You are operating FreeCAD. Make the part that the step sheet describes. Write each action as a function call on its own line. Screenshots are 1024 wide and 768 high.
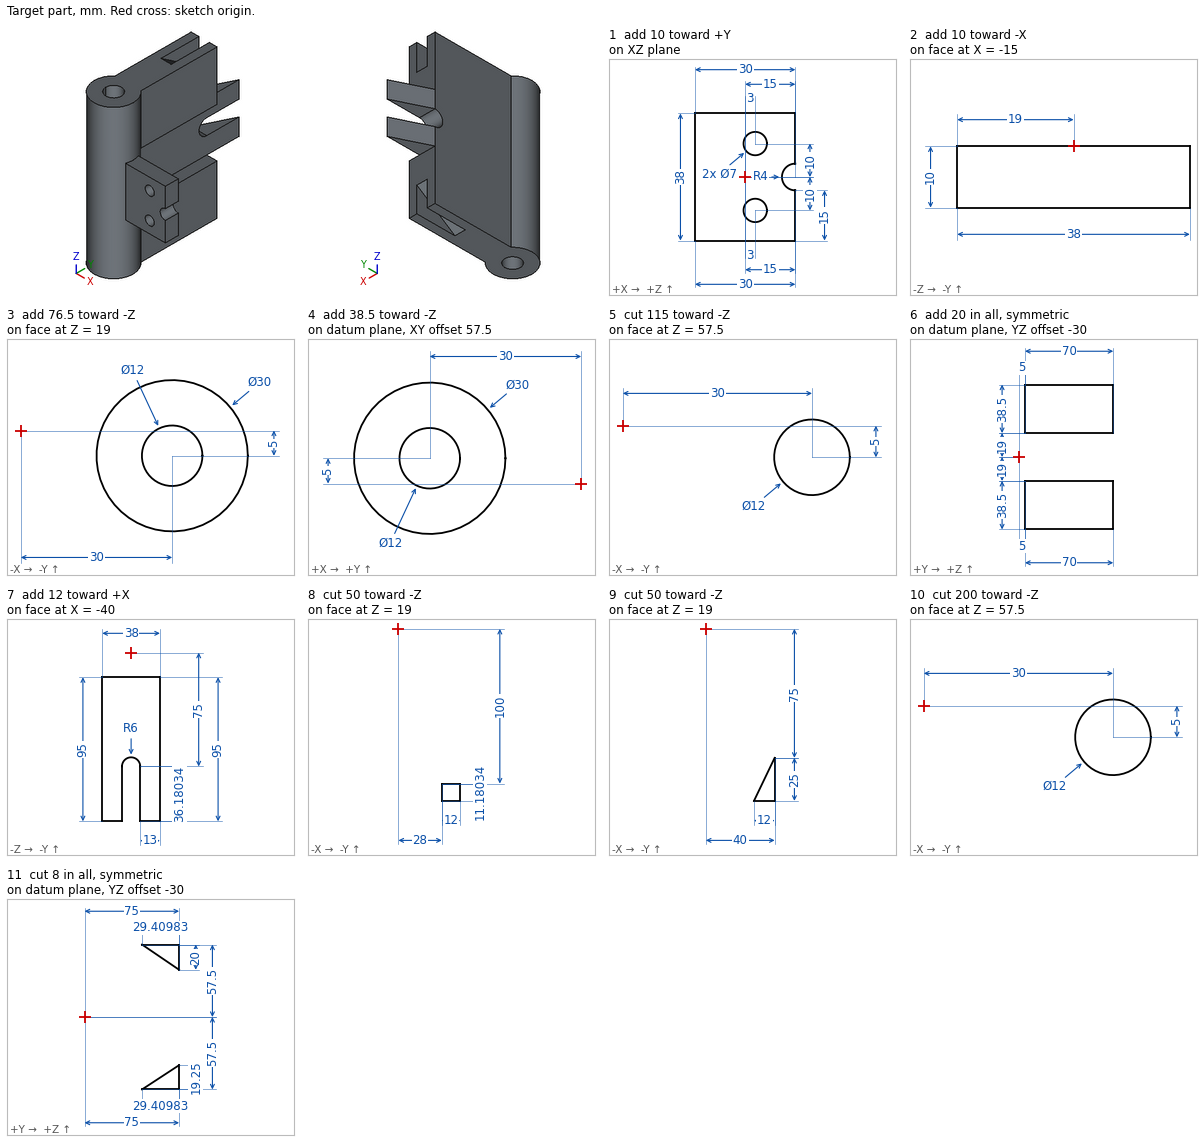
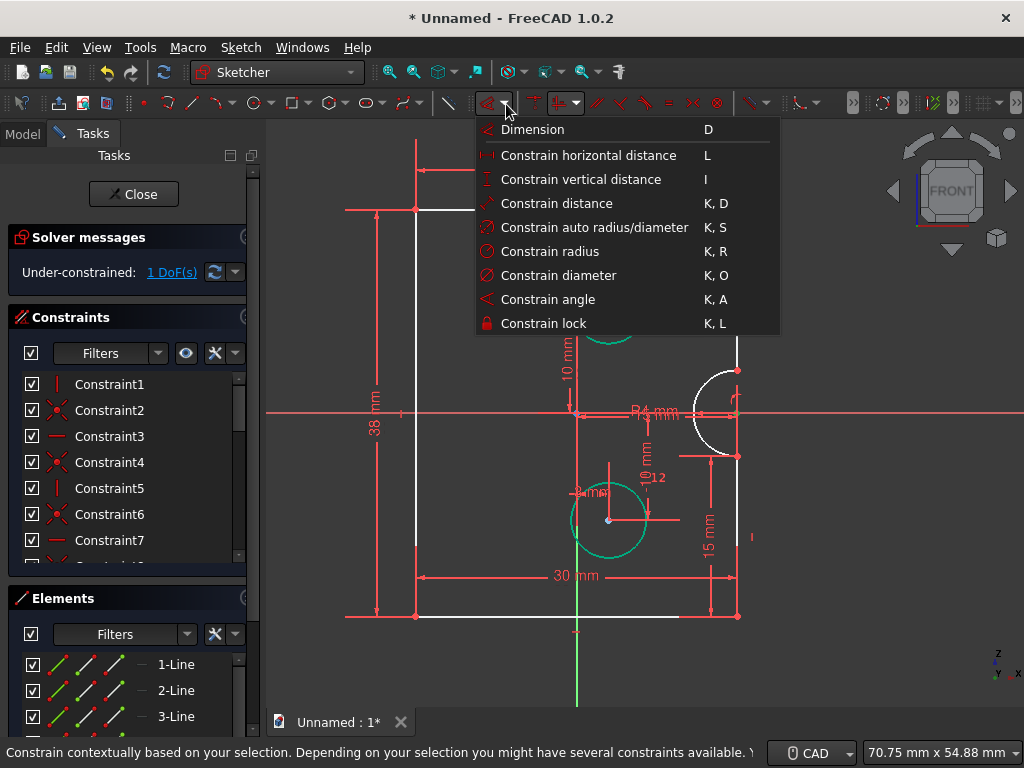
click(628, 155)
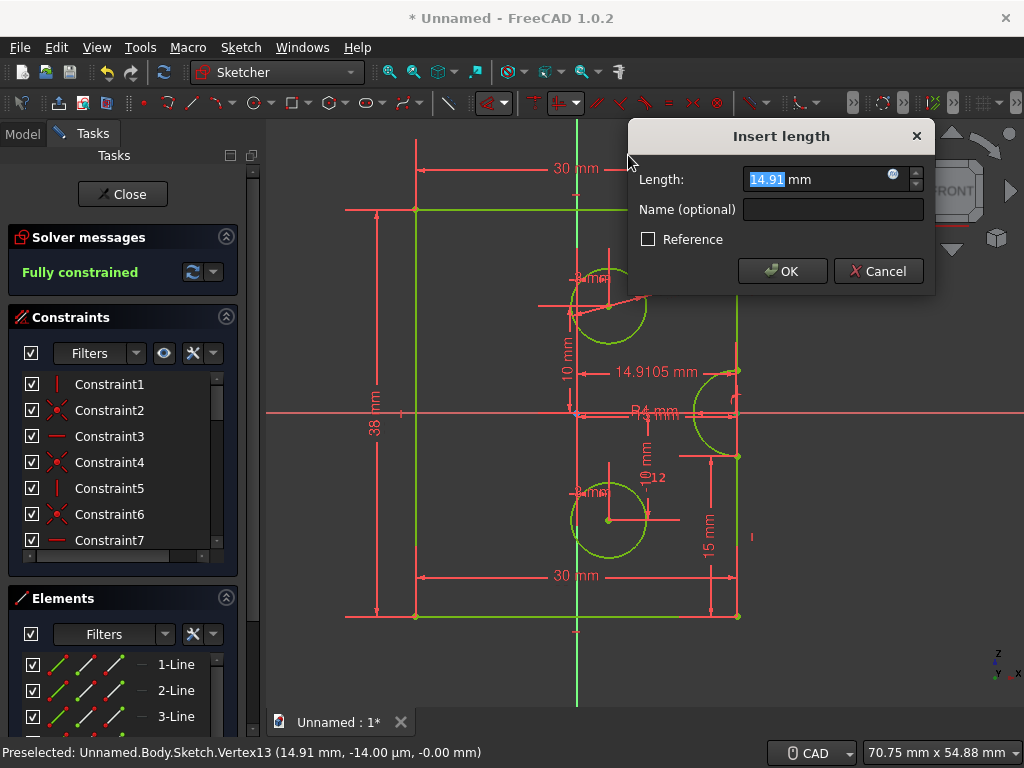
text(15)
key(Return)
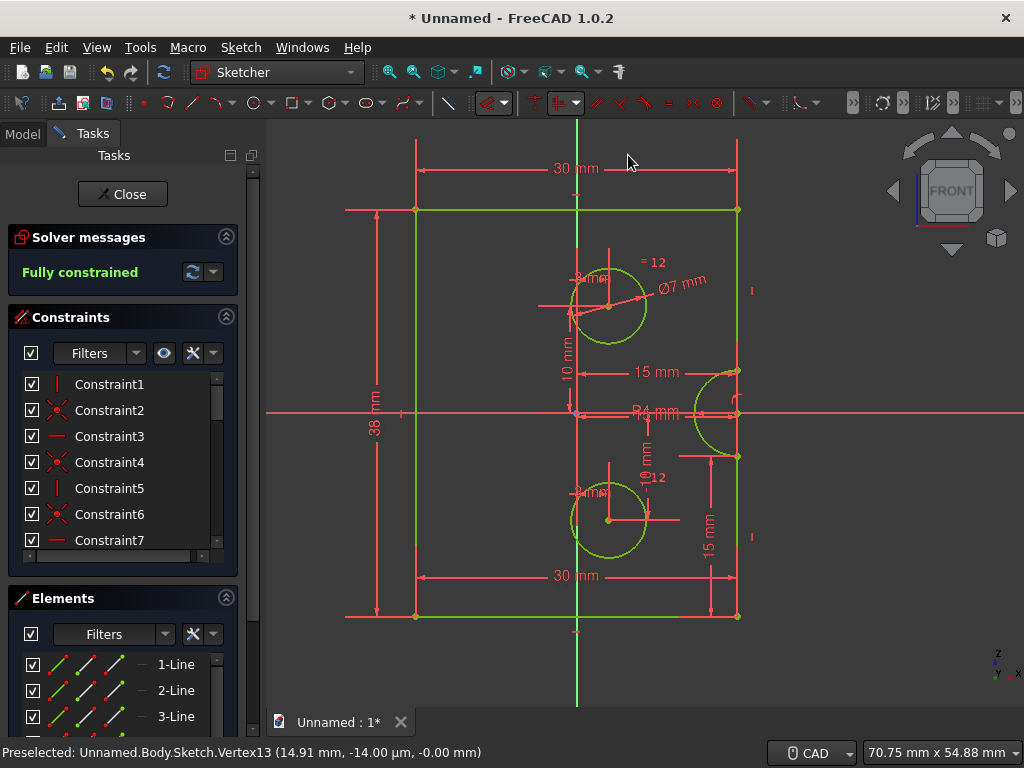
click(123, 194)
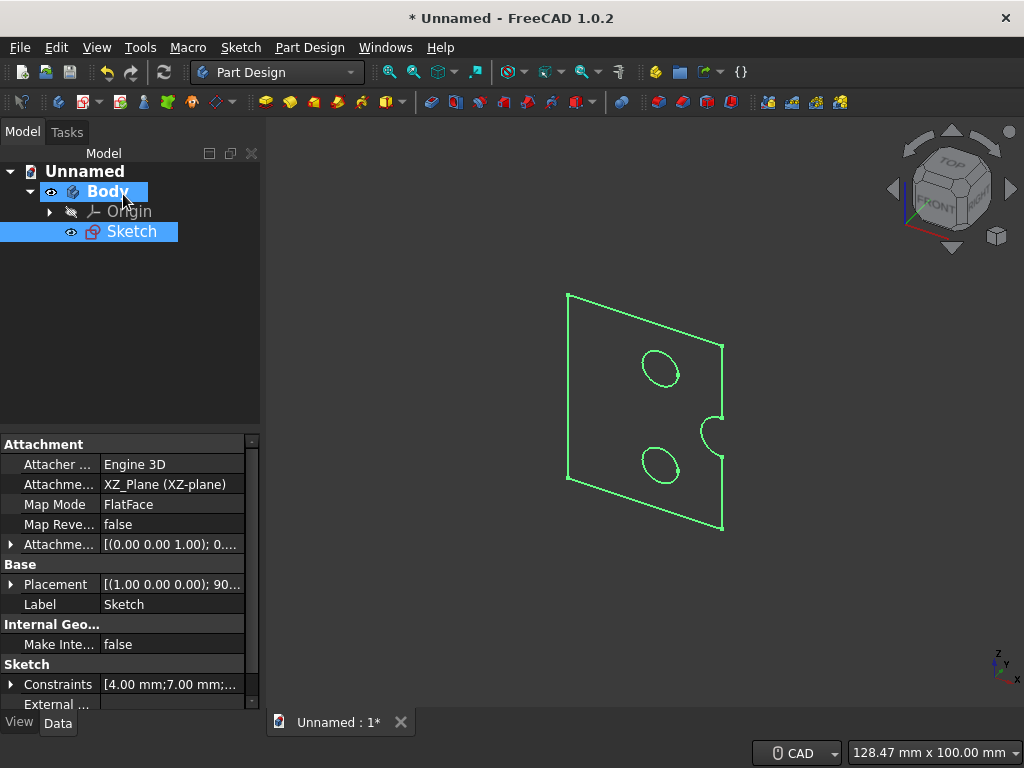
click(266, 102)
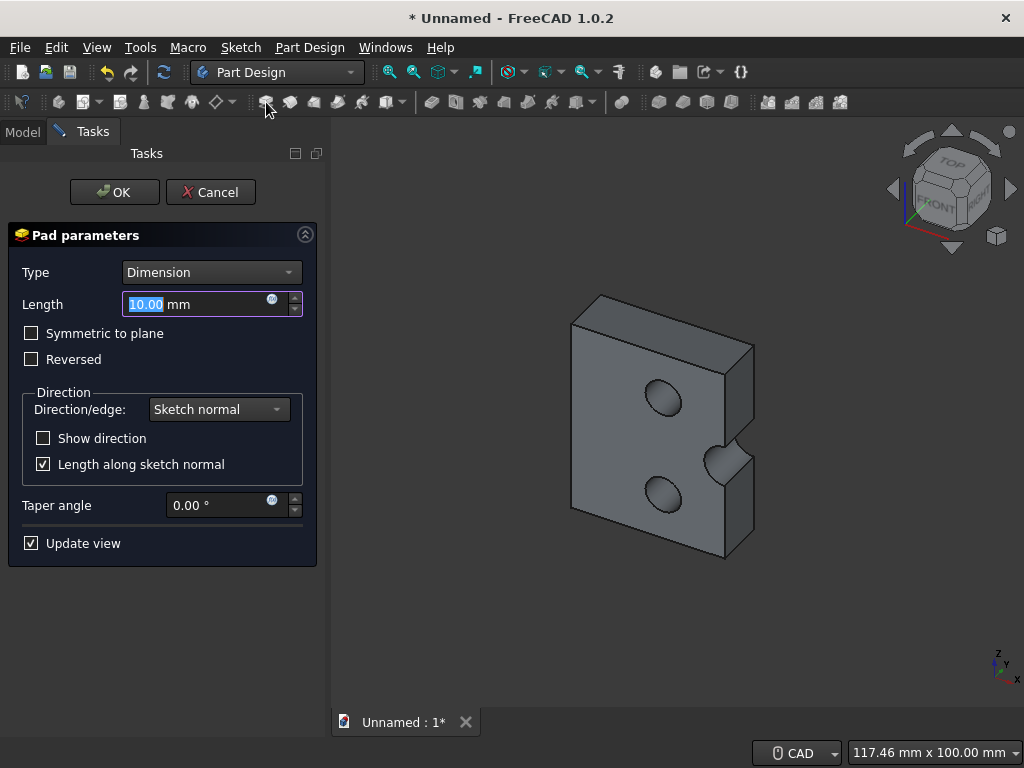
text(10)
key(Tab)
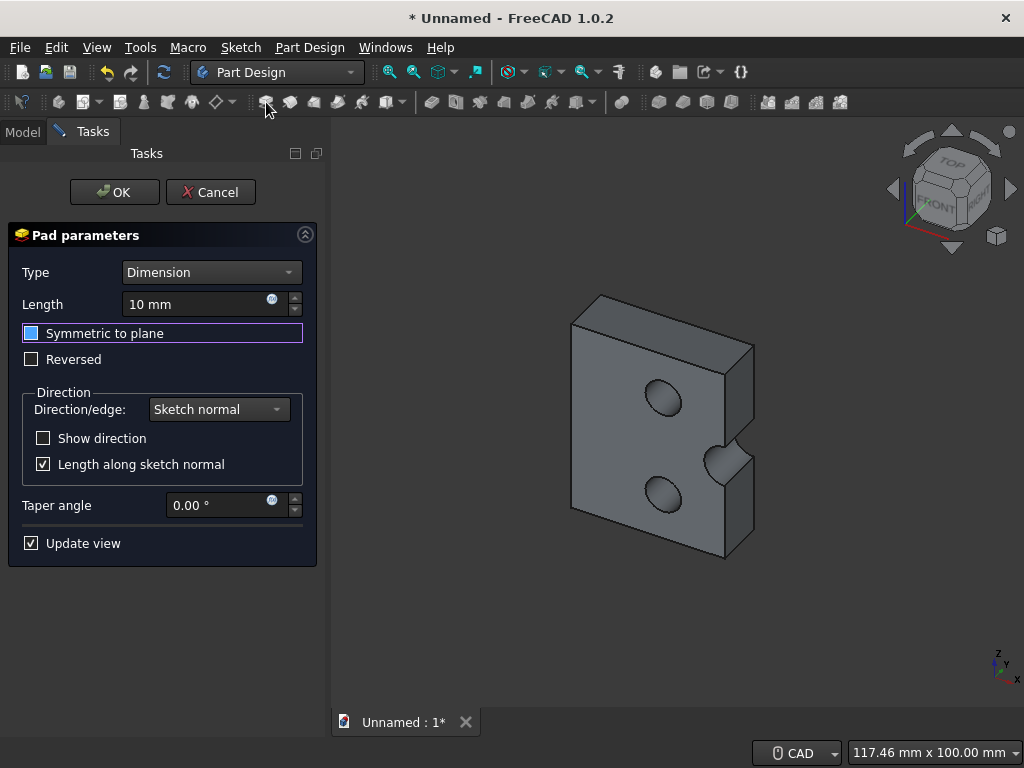
click(30, 359)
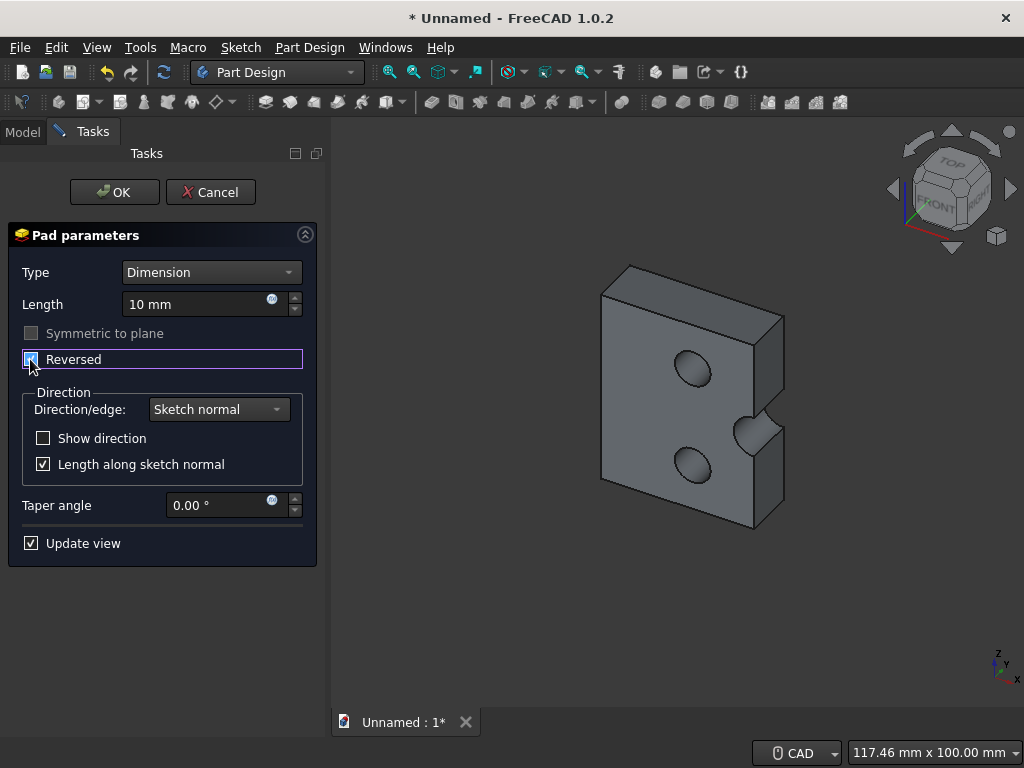
click(115, 192)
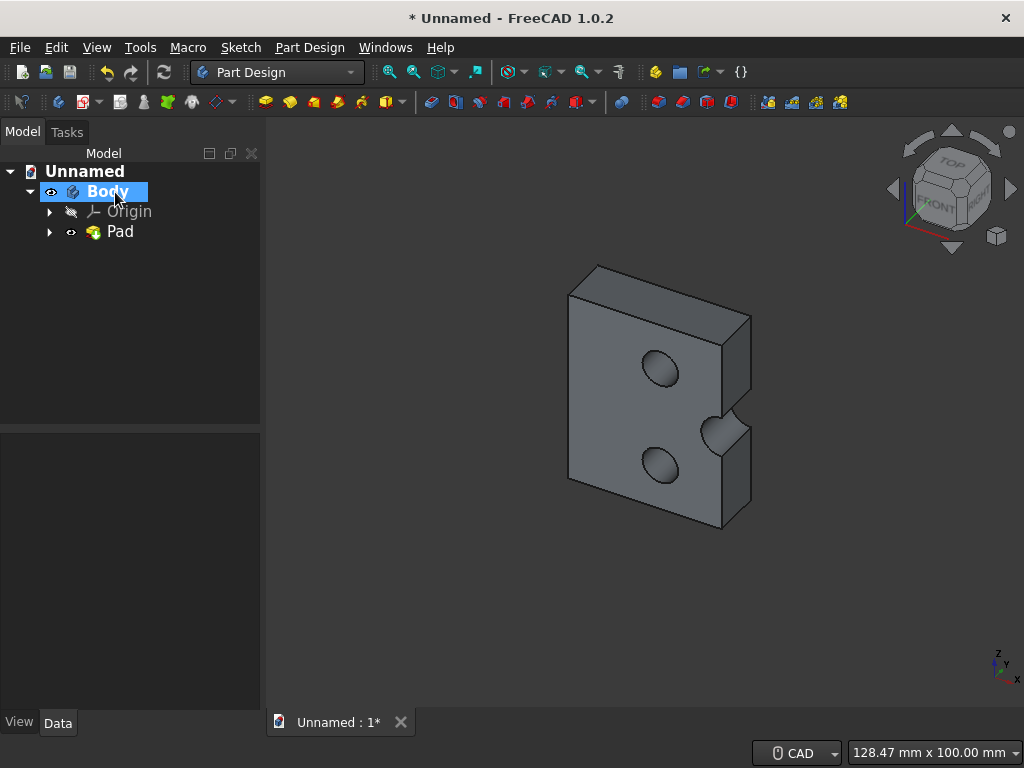
key(v)
key(f)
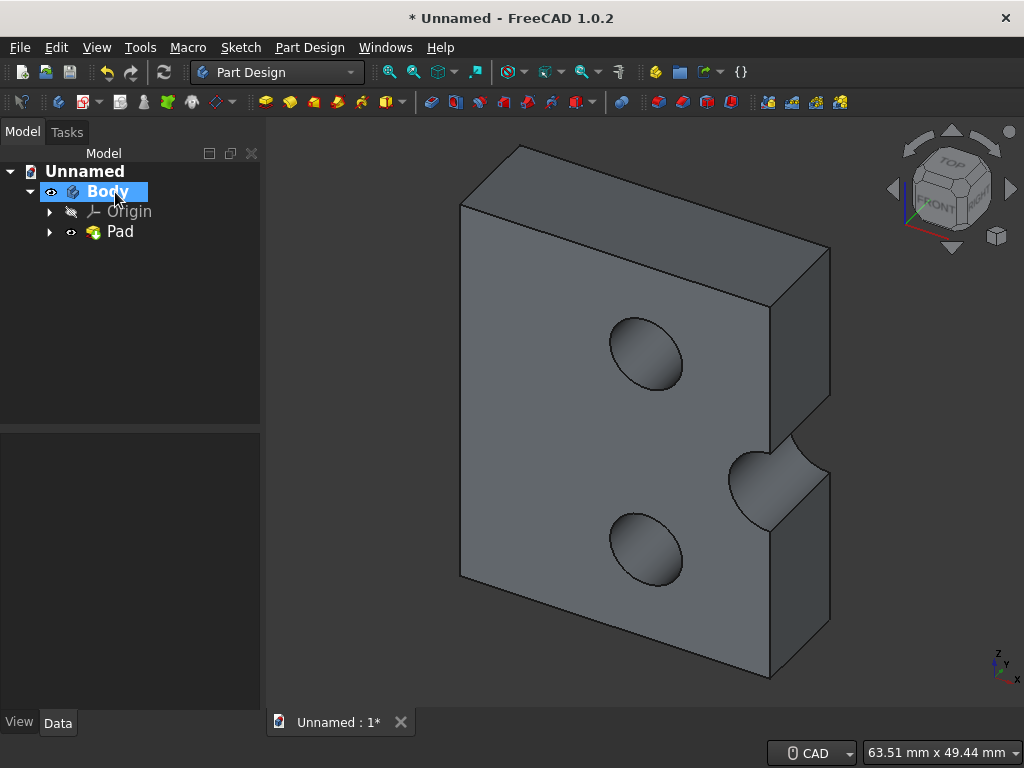
key(6)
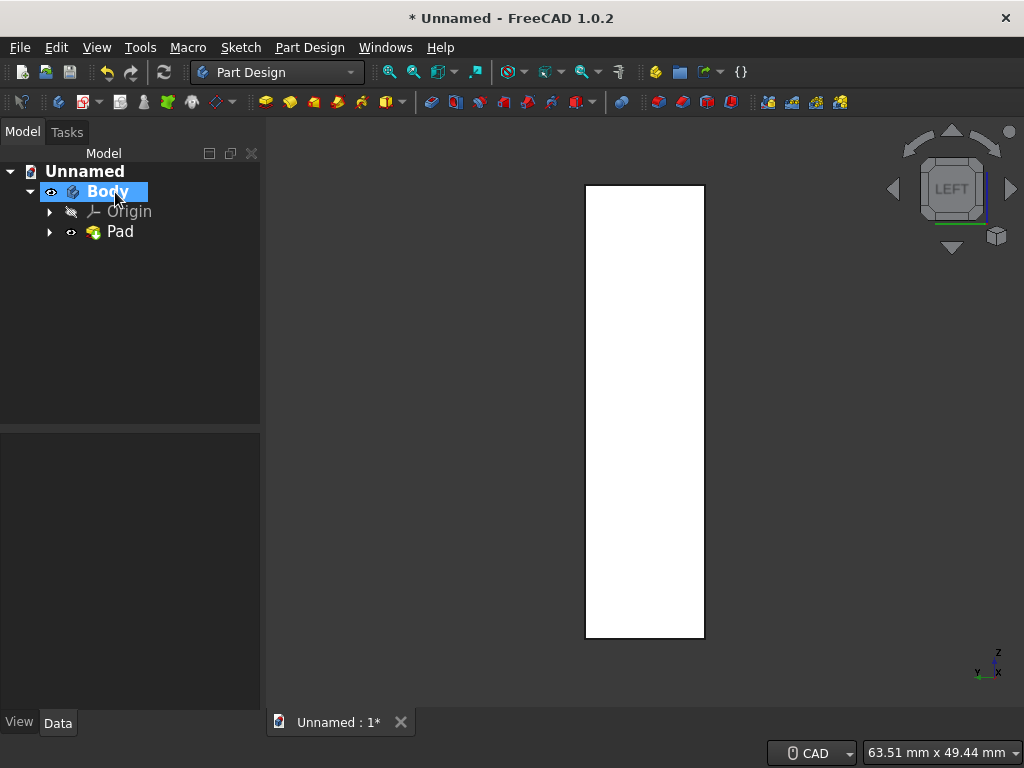
click(645, 346)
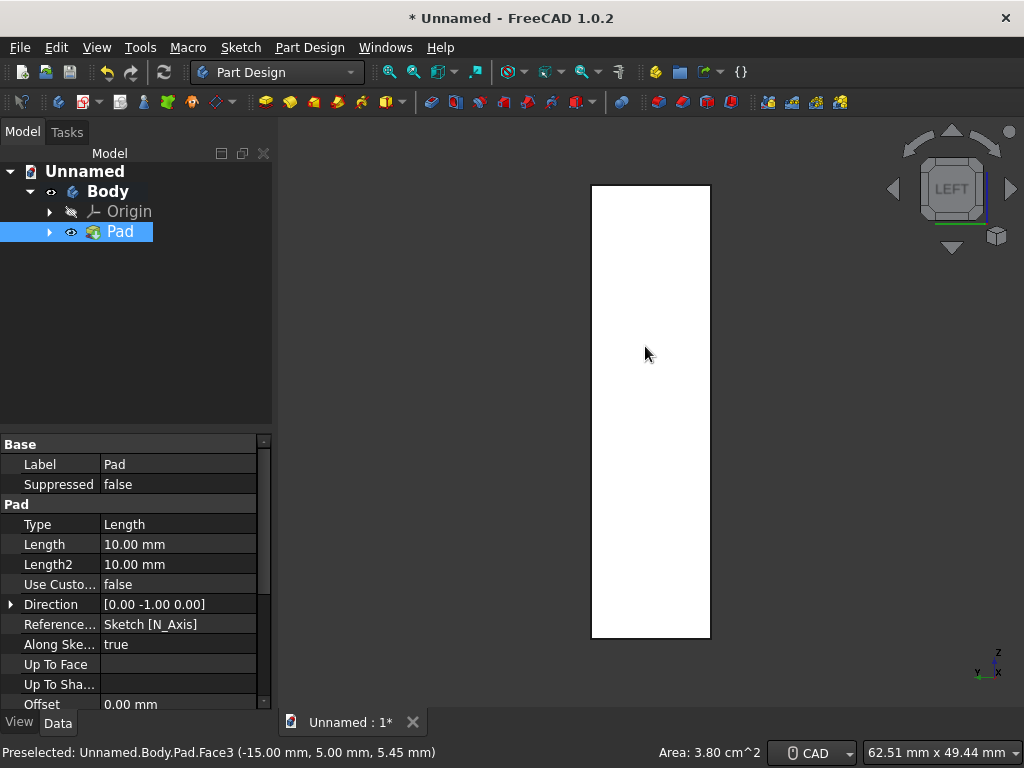
click(84, 102)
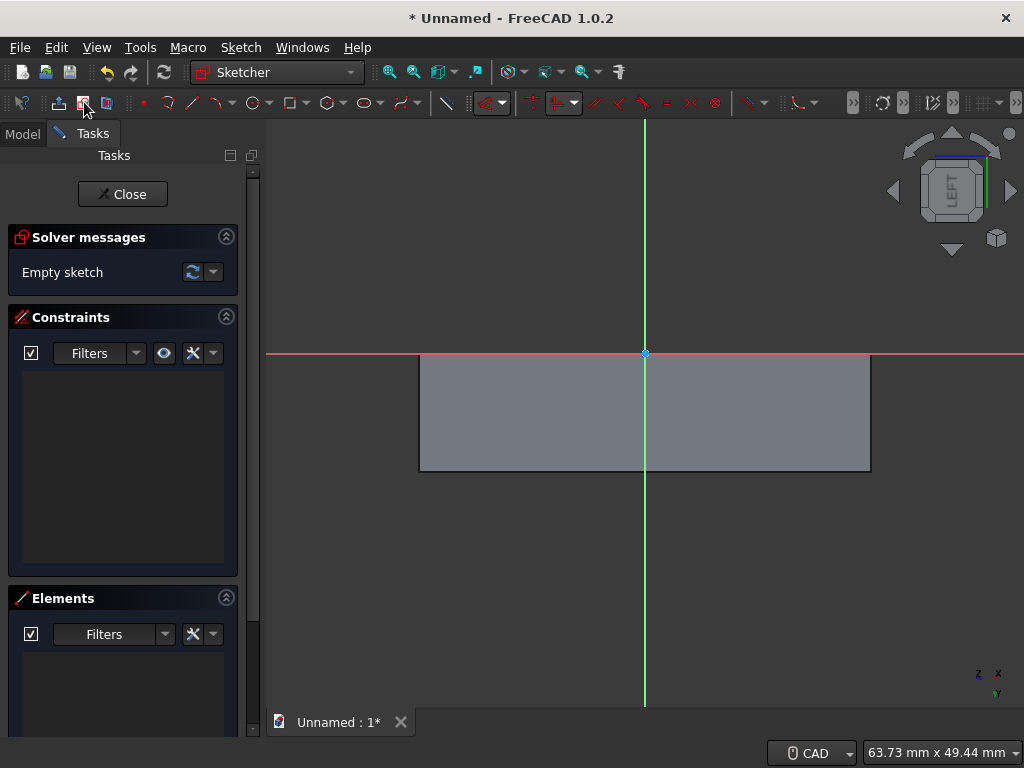
scroll(294, 413, down, 1)